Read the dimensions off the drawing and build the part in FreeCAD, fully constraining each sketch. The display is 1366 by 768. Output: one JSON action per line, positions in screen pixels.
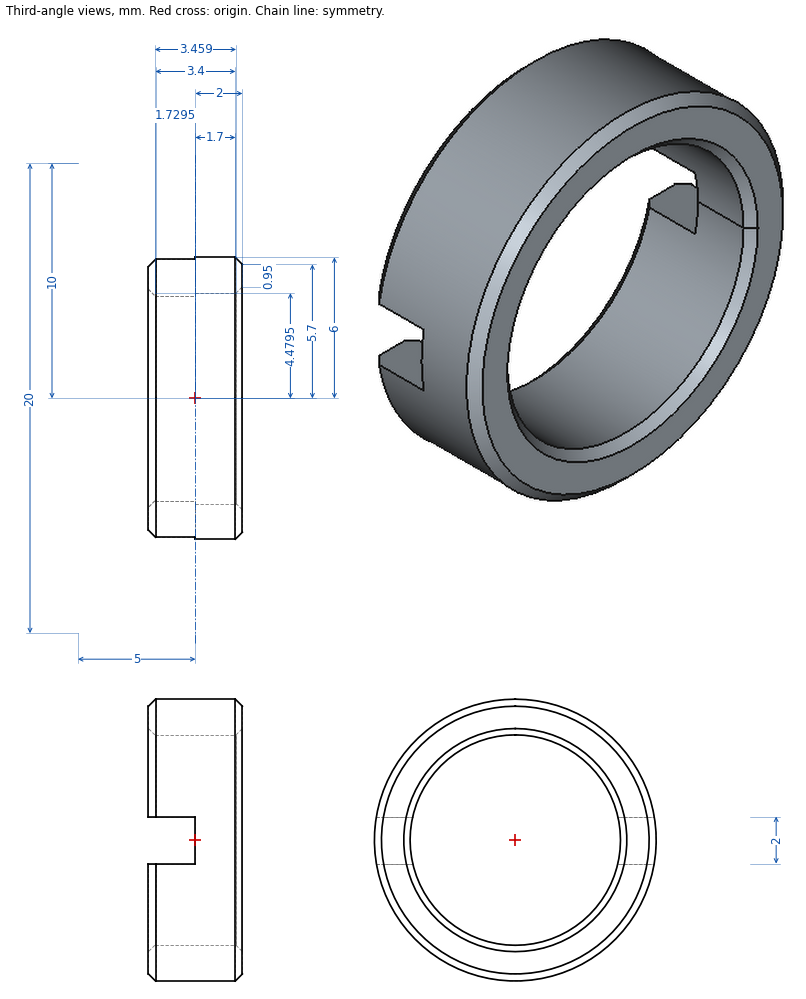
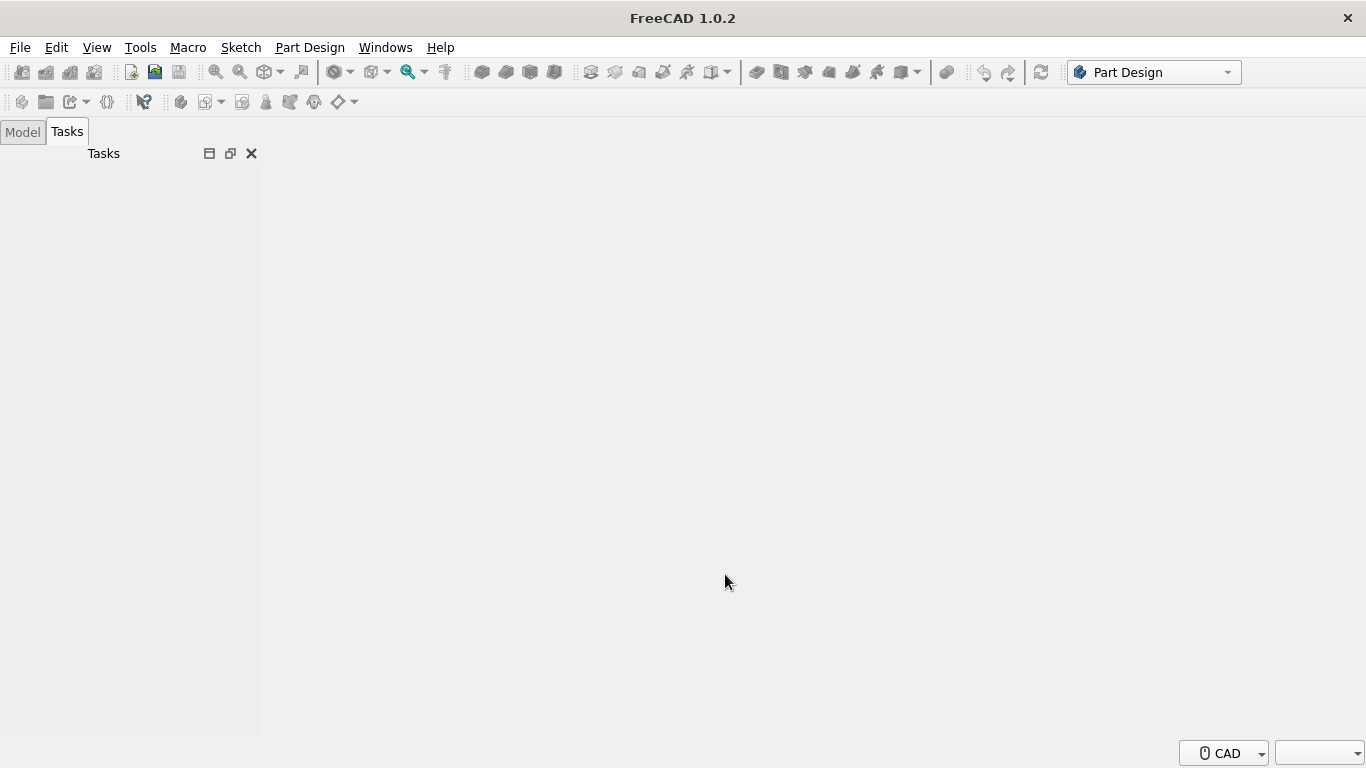
{"action": "left_click", "coordinate": [132, 72]}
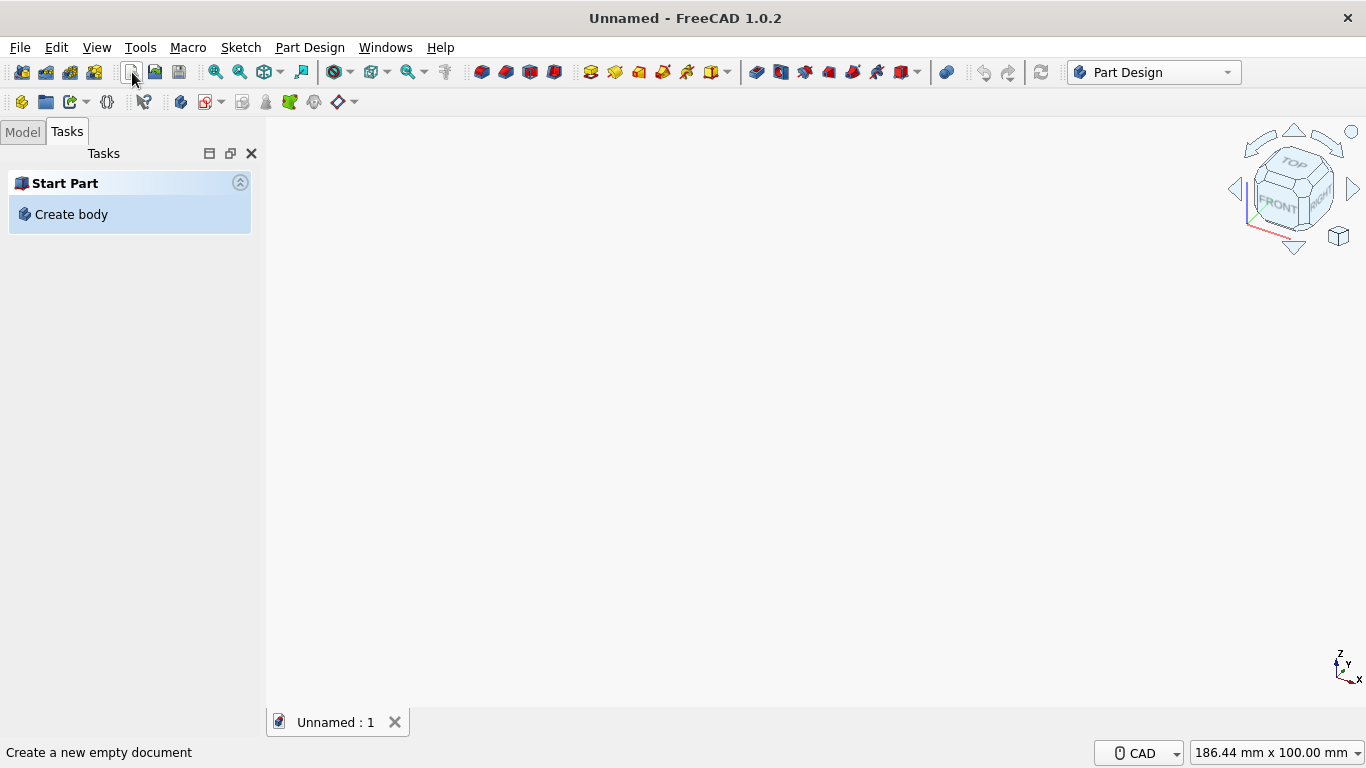
{"action": "left_click", "coordinate": [206, 102]}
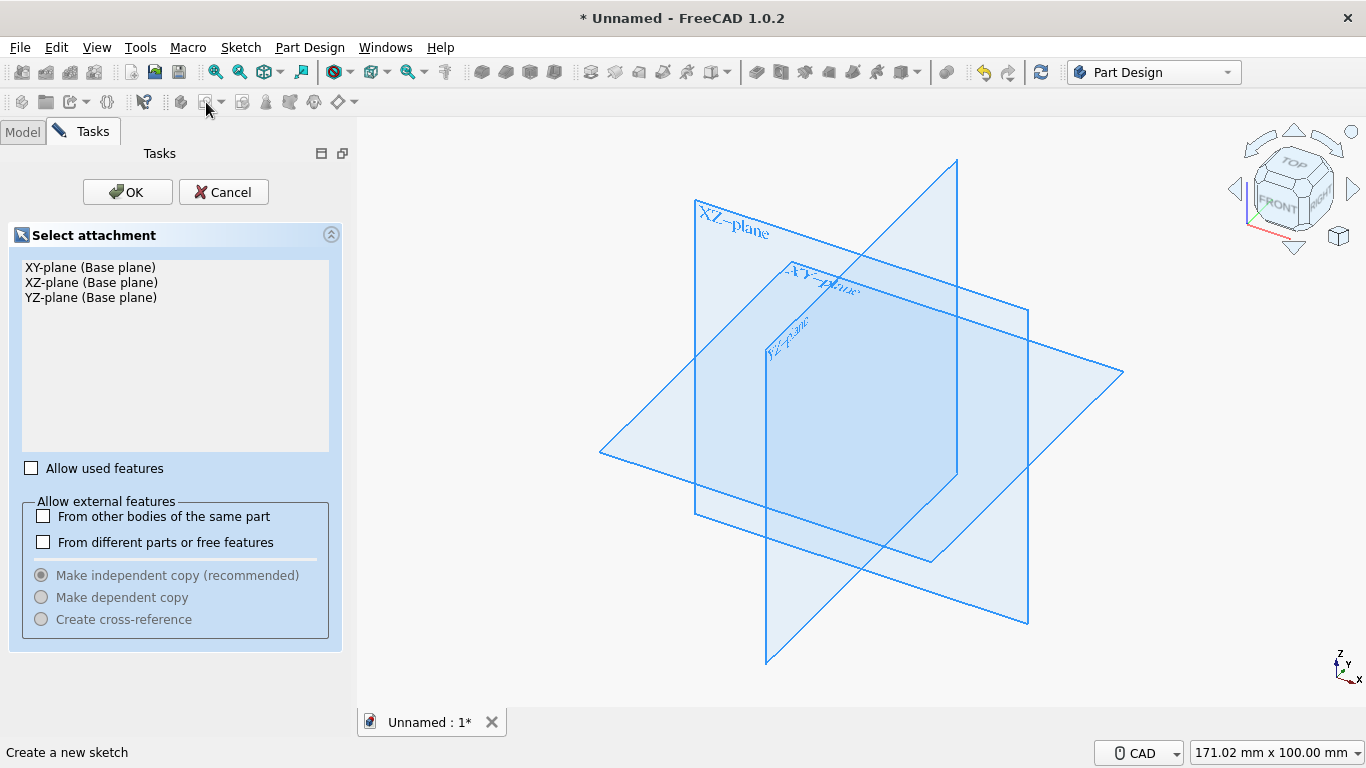
{"action": "left_click", "coordinate": [82, 268]}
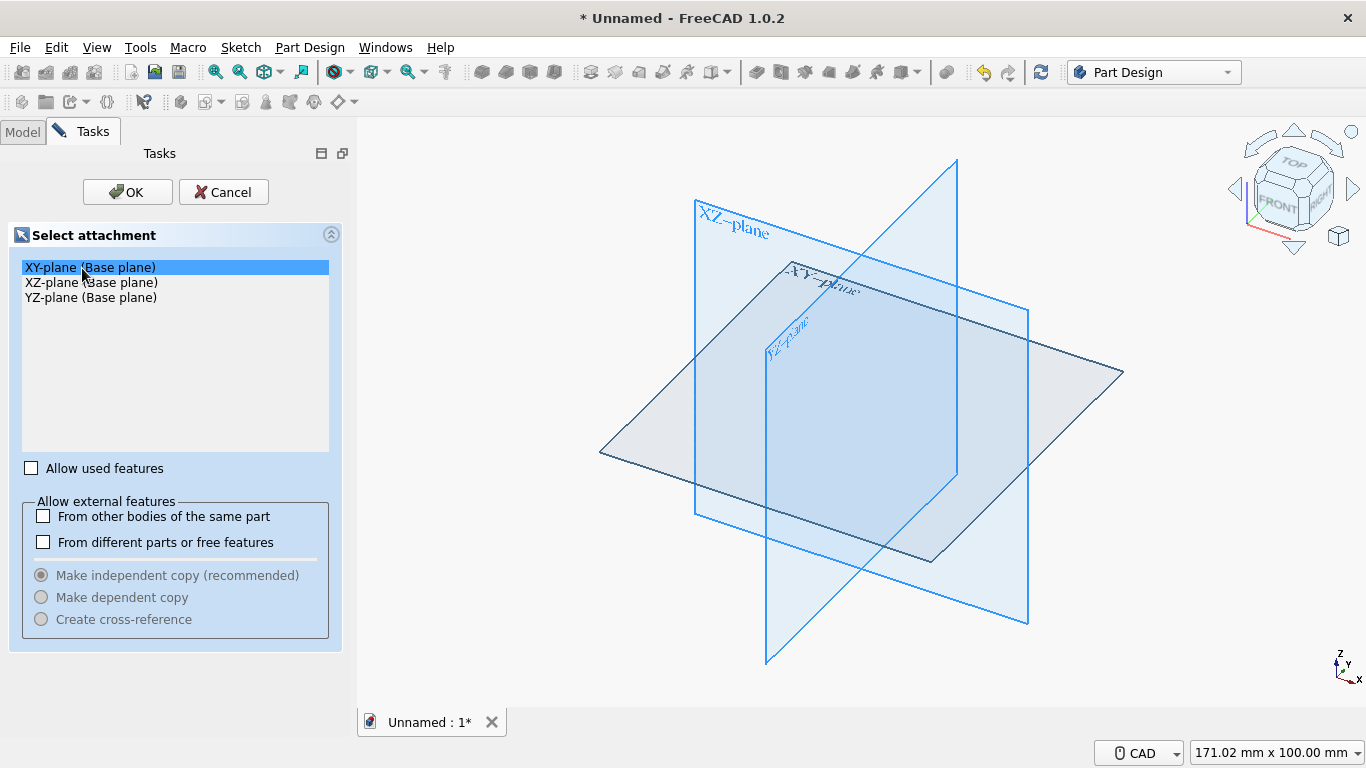
{"action": "left_click", "coordinate": [128, 192]}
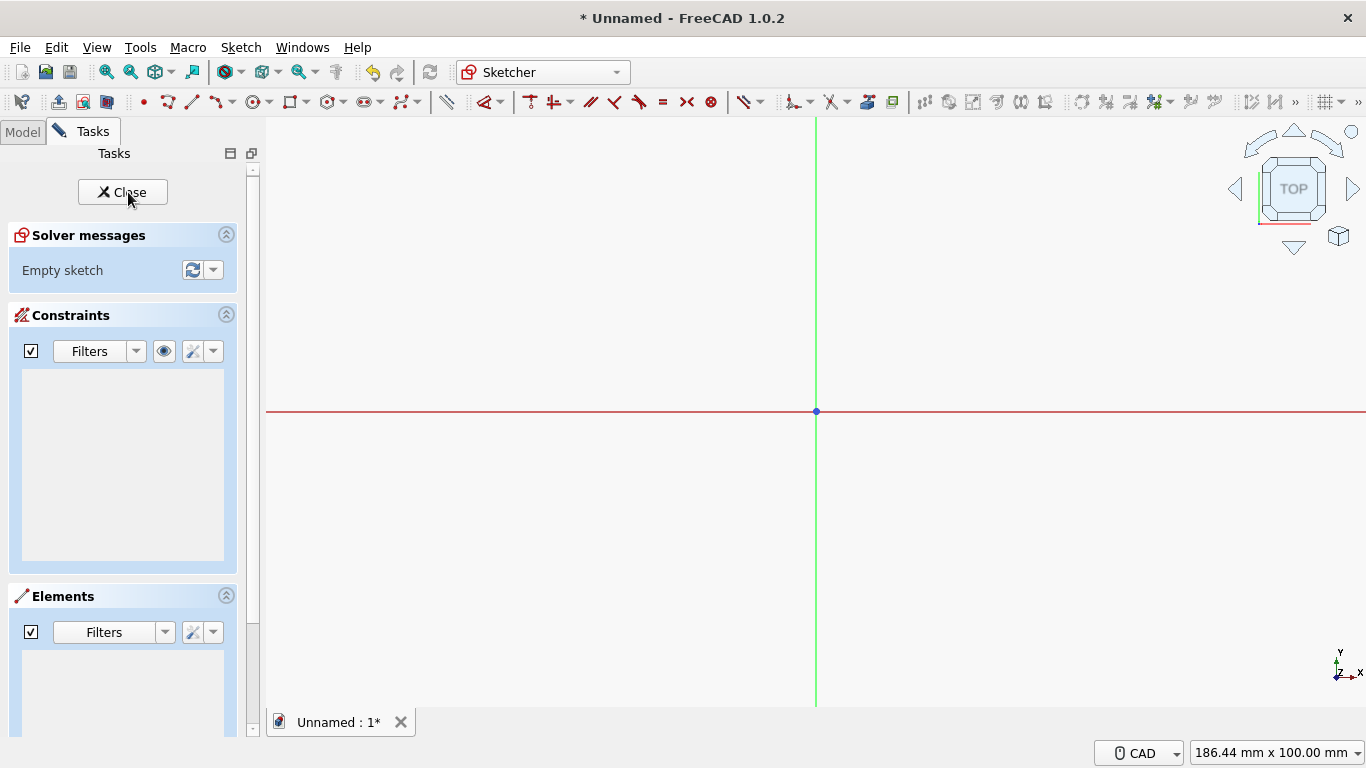
{"action": "scroll", "coordinate": [823, 393], "scroll_direction": "up", "scroll_amount": 12}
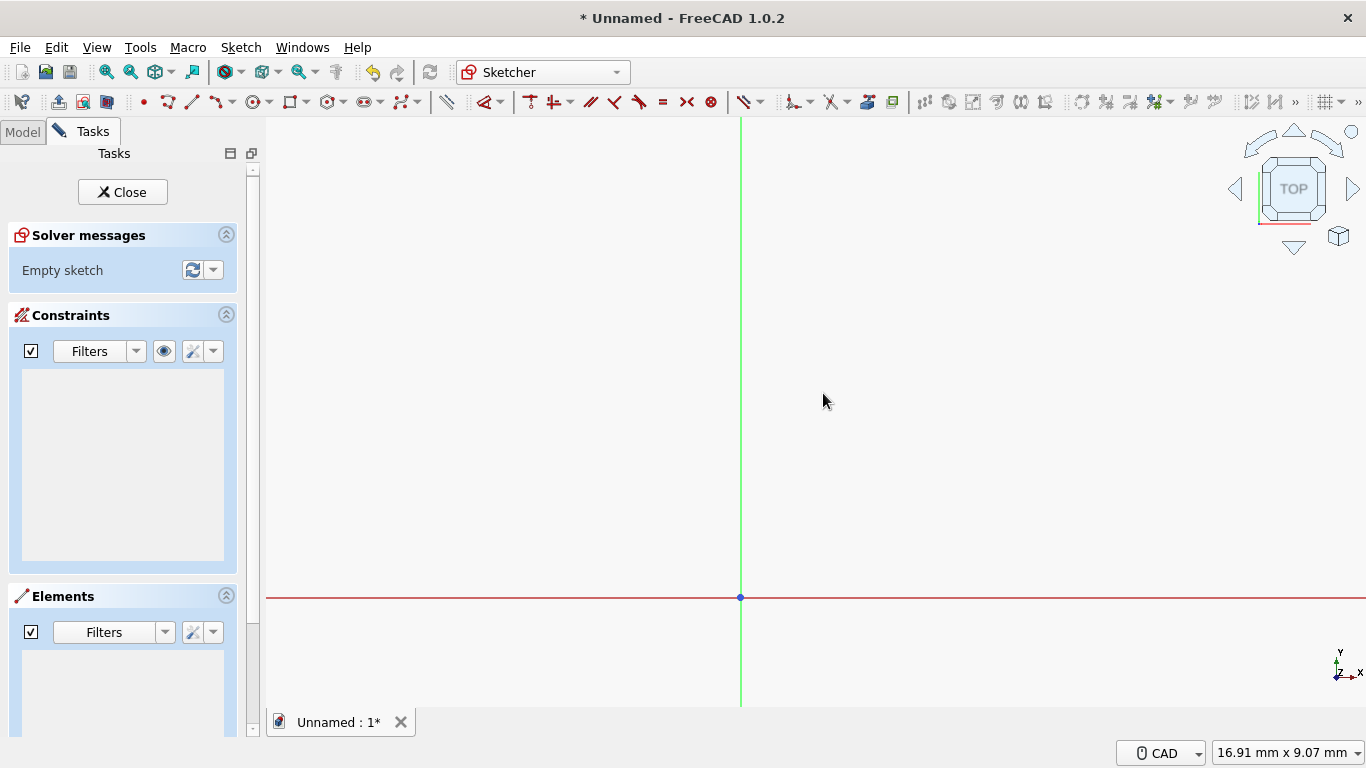
{"action": "left_click", "coordinate": [168, 102]}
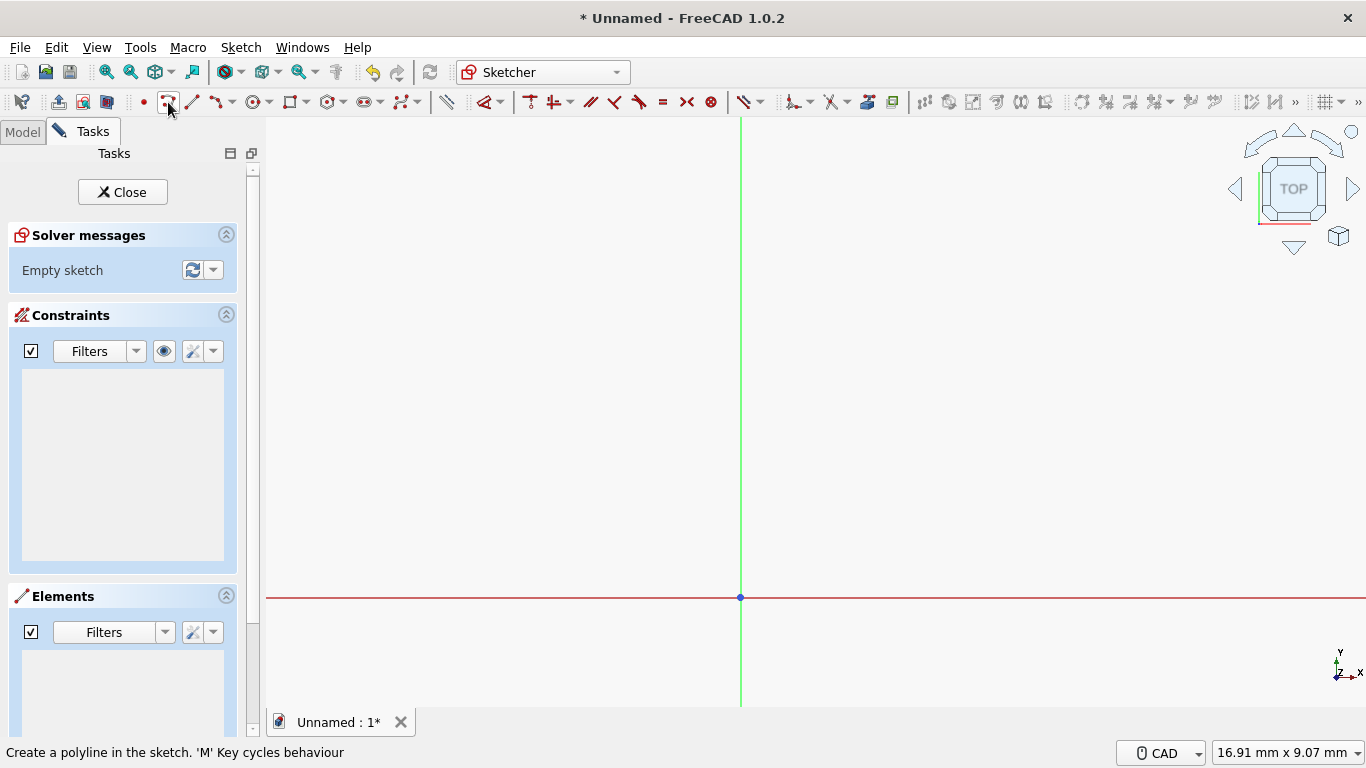
{"action": "left_click", "coordinate": [628, 306]}
{"action": "left_click", "coordinate": [853, 306]}
{"action": "left_click", "coordinate": [871, 289]}
{"action": "left_click", "coordinate": [871, 227]}
{"action": "left_click", "coordinate": [851, 208]}
{"action": "left_click", "coordinate": [630, 208]}
{"action": "left_click", "coordinate": [611, 227]}
{"action": "left_click", "coordinate": [611, 289]}
{"action": "left_click", "coordinate": [628, 307]}
{"action": "key", "text": "Escape"}
{"action": "key", "text": "Escape"}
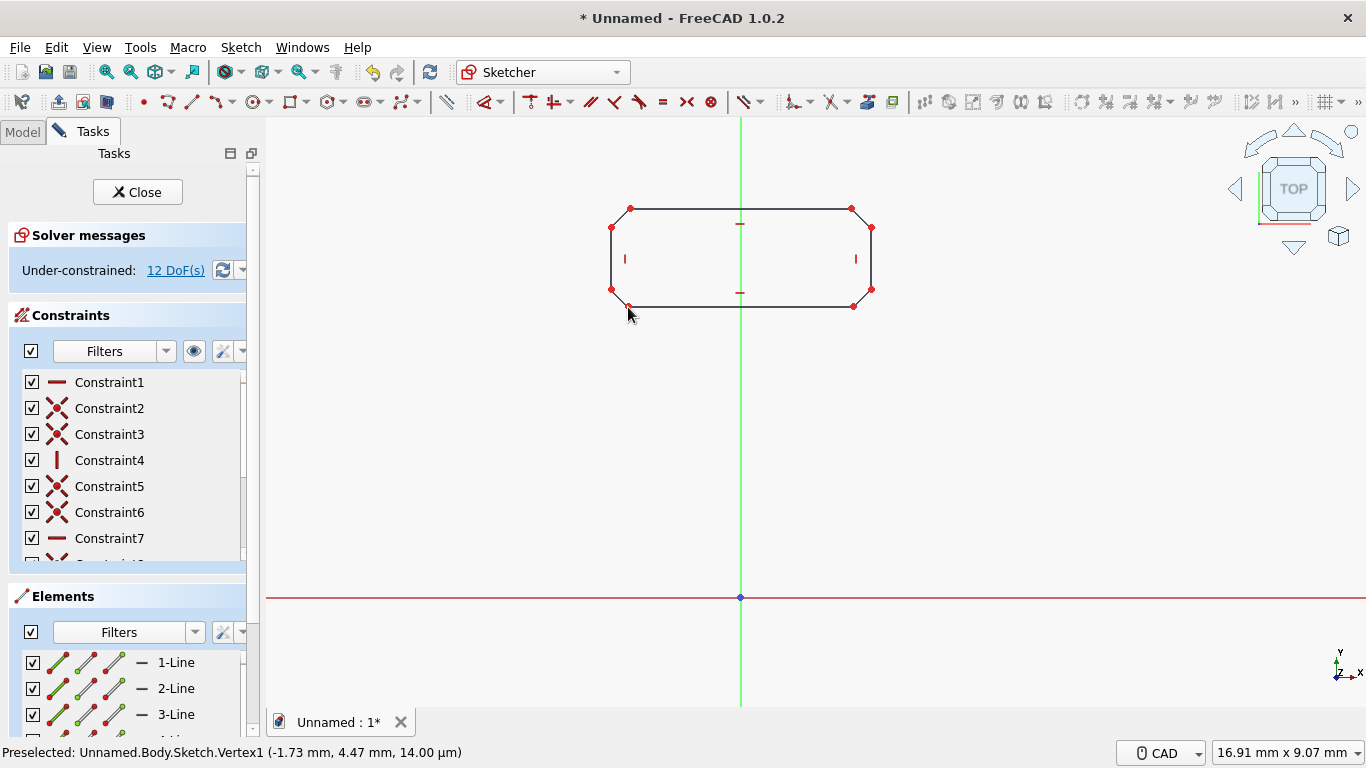
{"action": "left_click", "coordinate": [871, 228]}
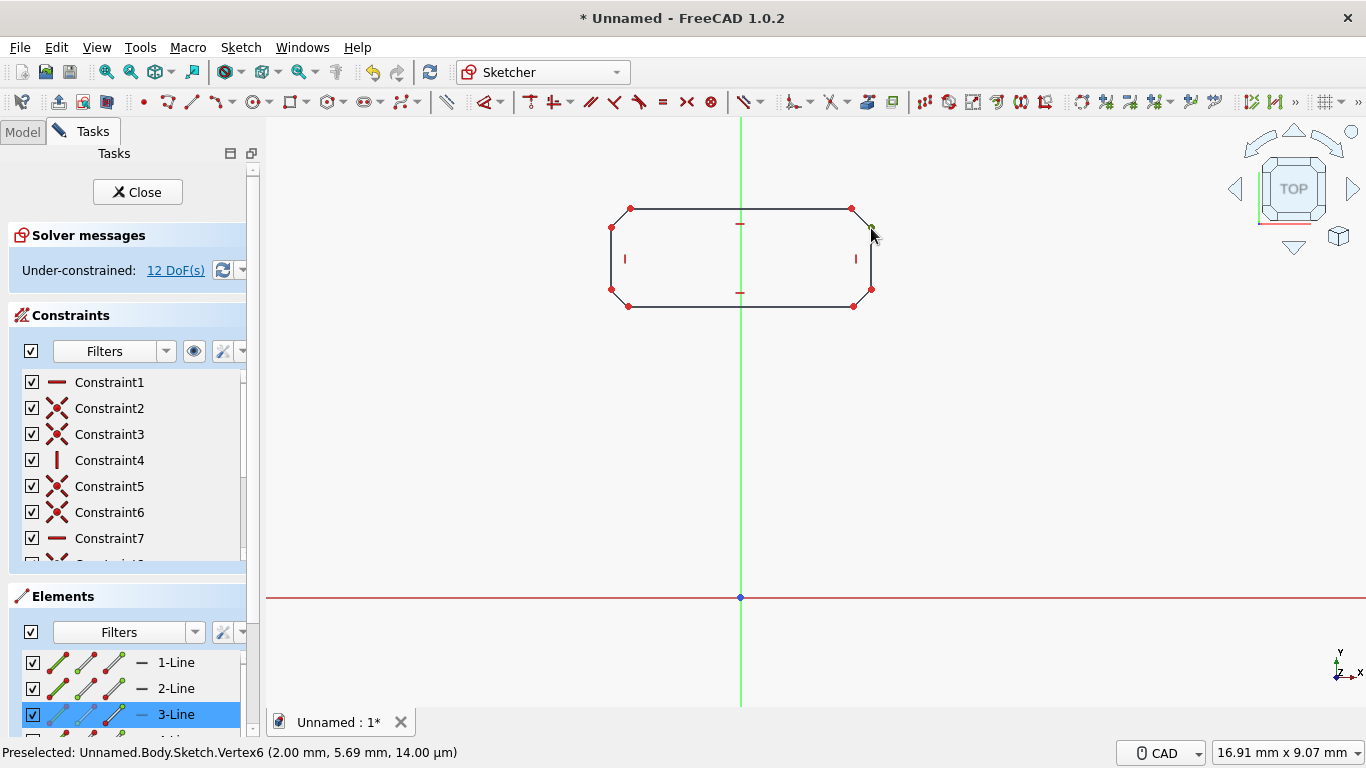
{"action": "left_click", "coordinate": [611, 228]}